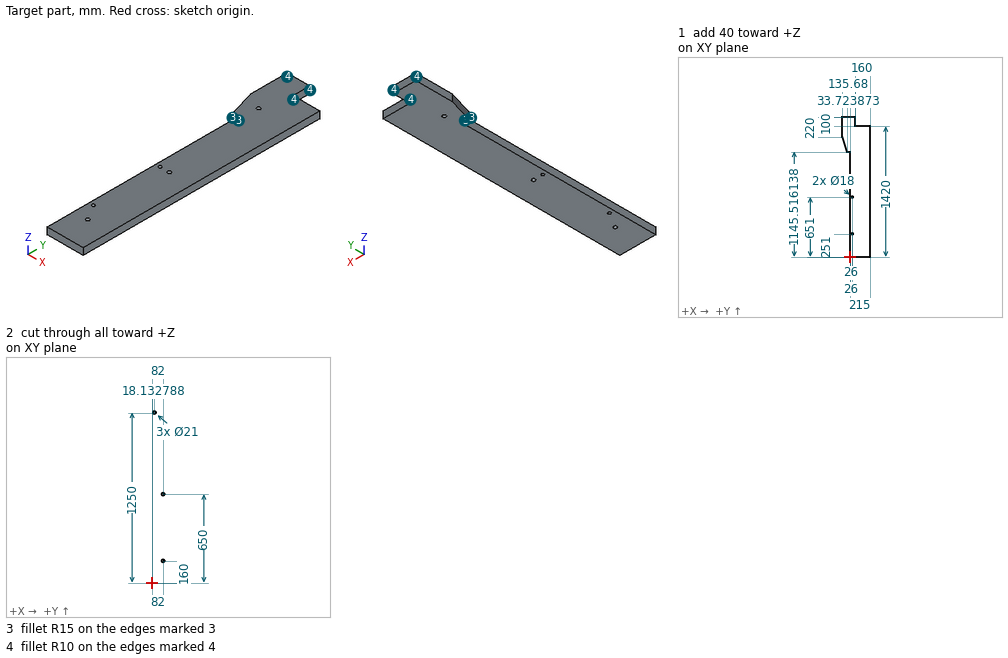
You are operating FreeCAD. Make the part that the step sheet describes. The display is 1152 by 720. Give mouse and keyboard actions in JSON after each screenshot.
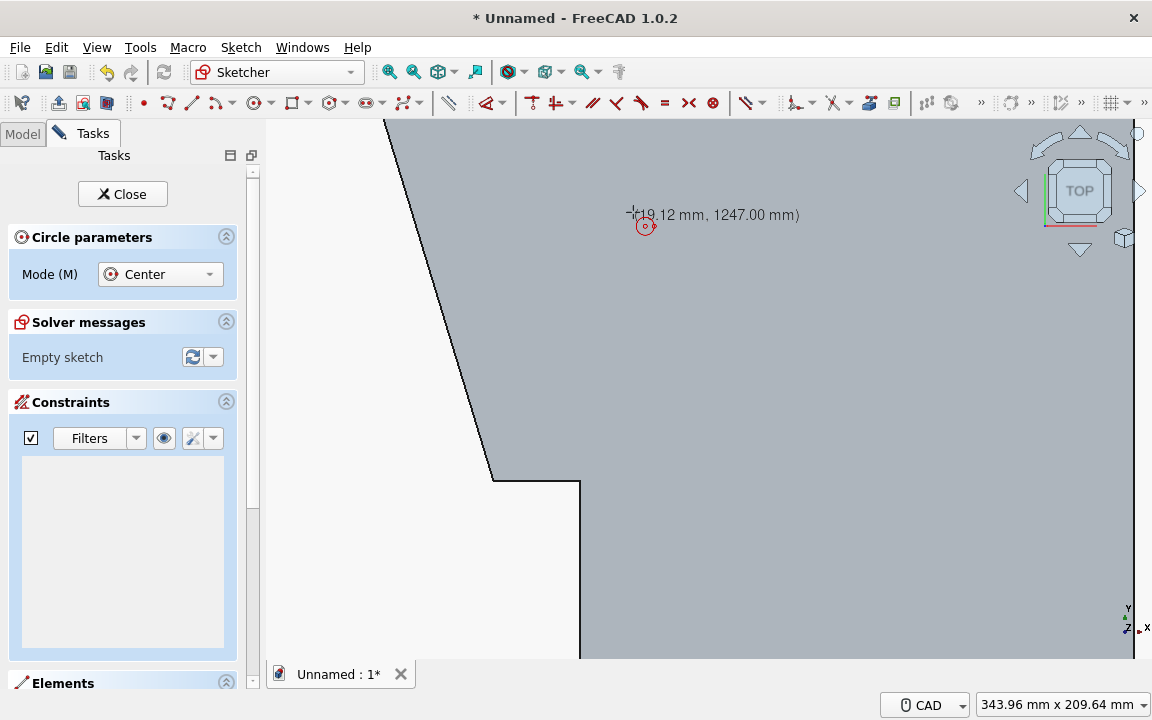
{"action": "scroll", "coordinate": [633, 212], "scroll_direction": "down", "scroll_amount": 11}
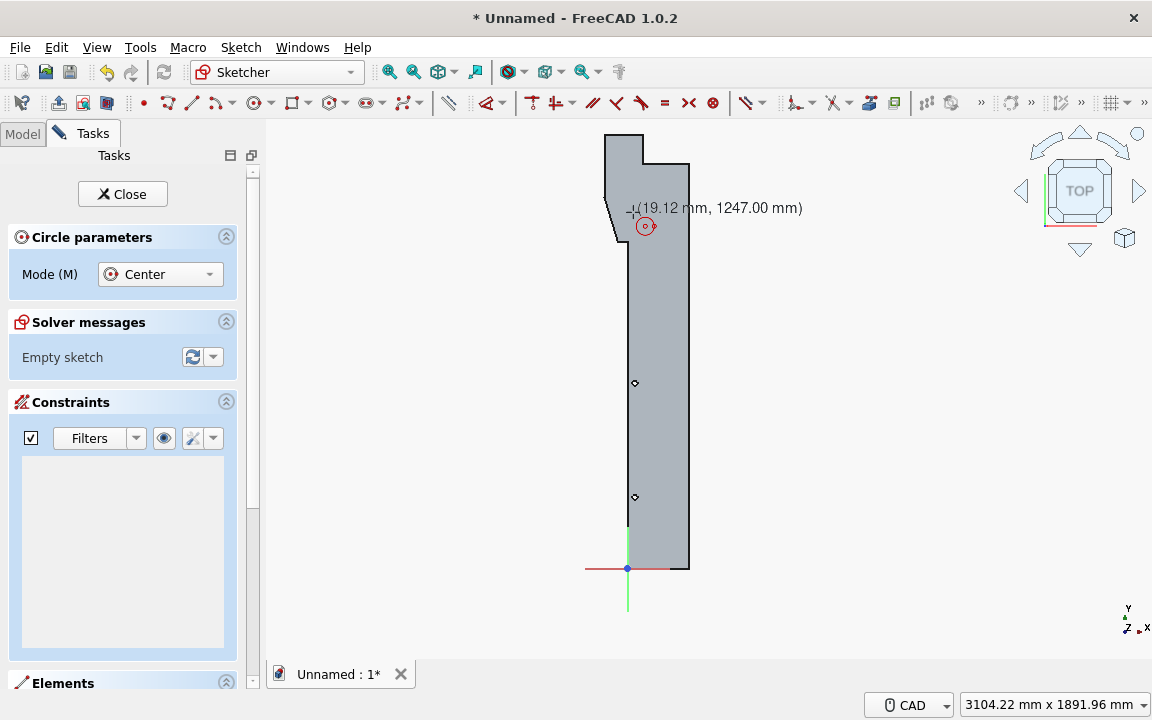
{"action": "scroll", "coordinate": [633, 212], "scroll_direction": "up", "scroll_amount": 6}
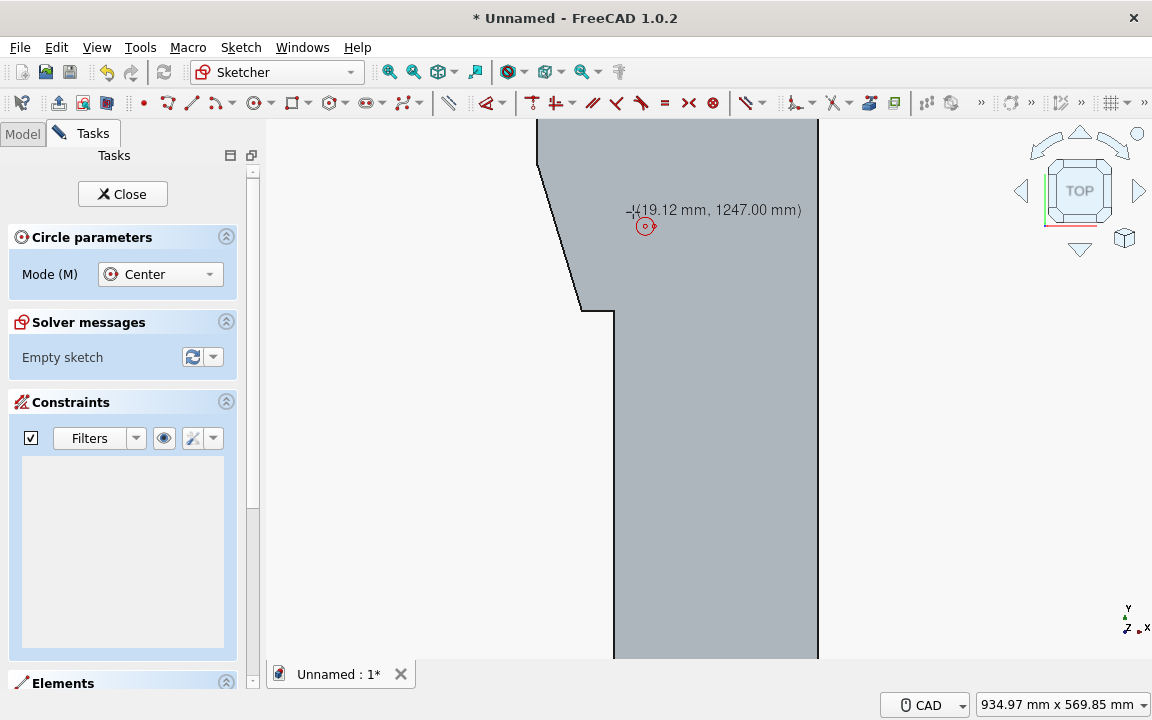
{"action": "left_click", "coordinate": [631, 212]}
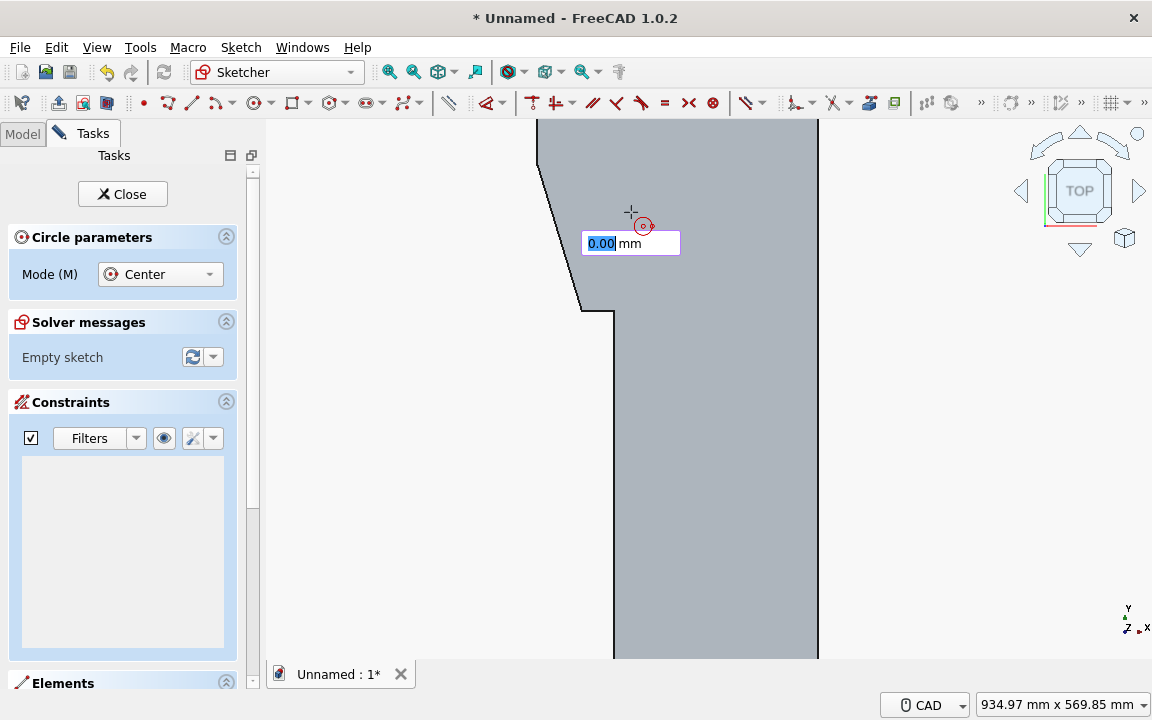
{"action": "scroll", "coordinate": [638, 205], "scroll_direction": "up", "scroll_amount": 3}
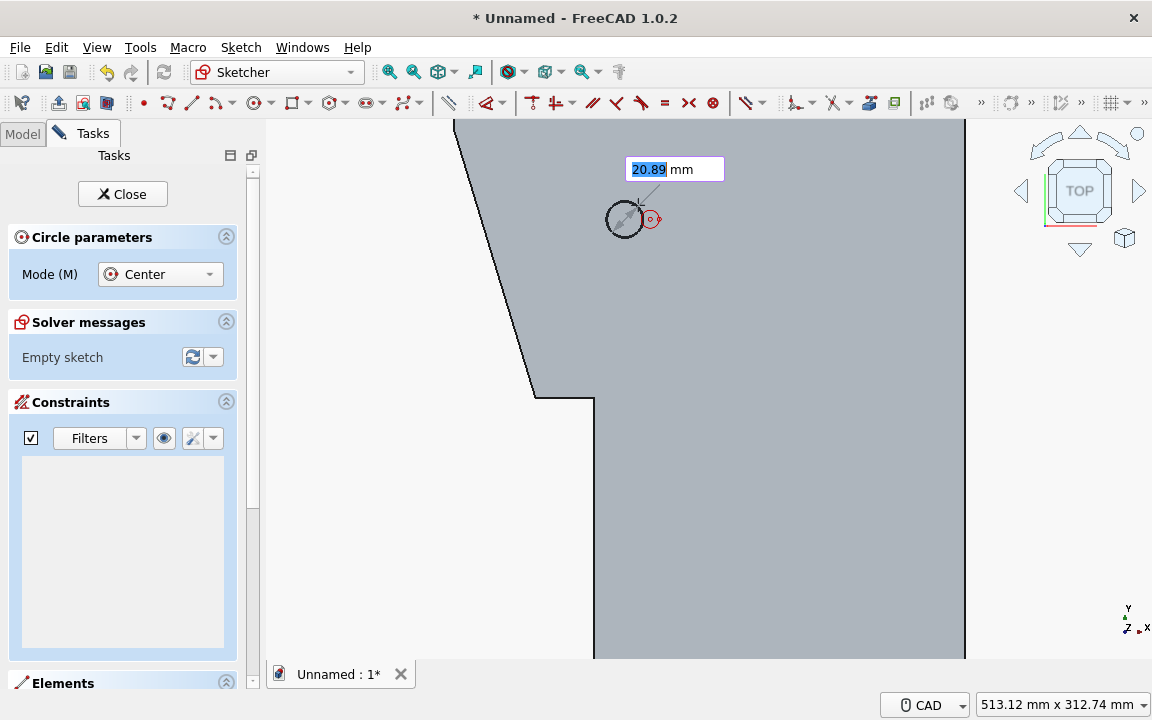
{"action": "left_click", "coordinate": [638, 205]}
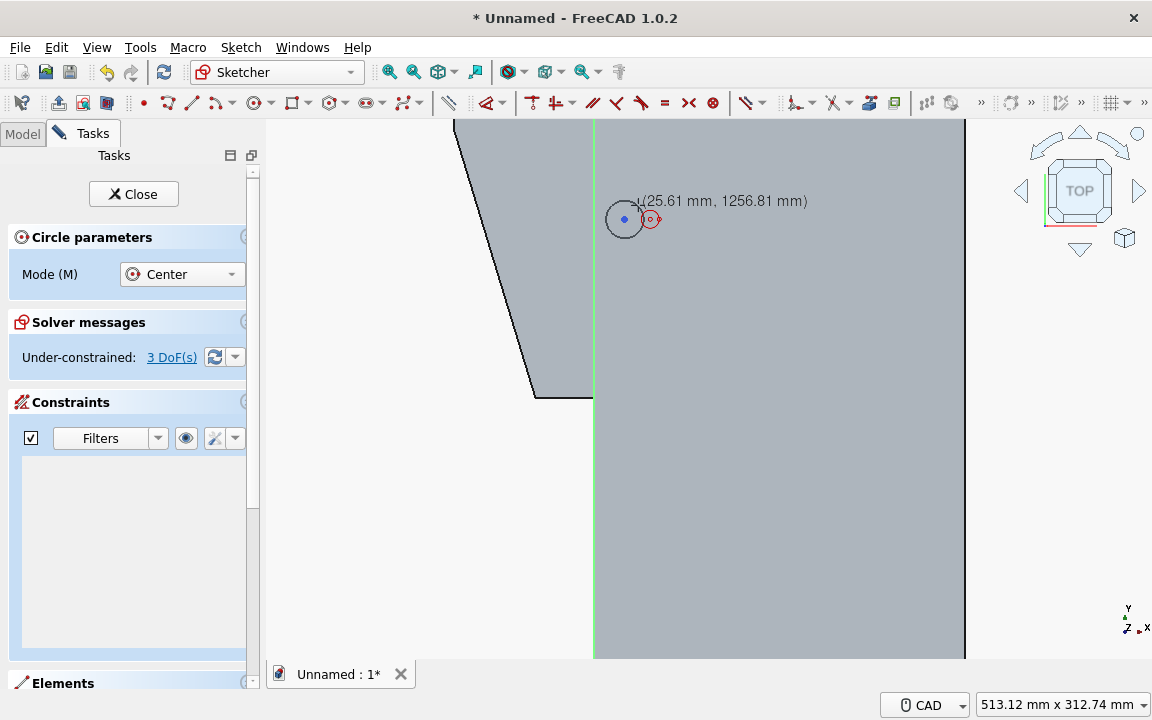
{"action": "scroll", "coordinate": [634, 211], "scroll_direction": "down", "scroll_amount": 9}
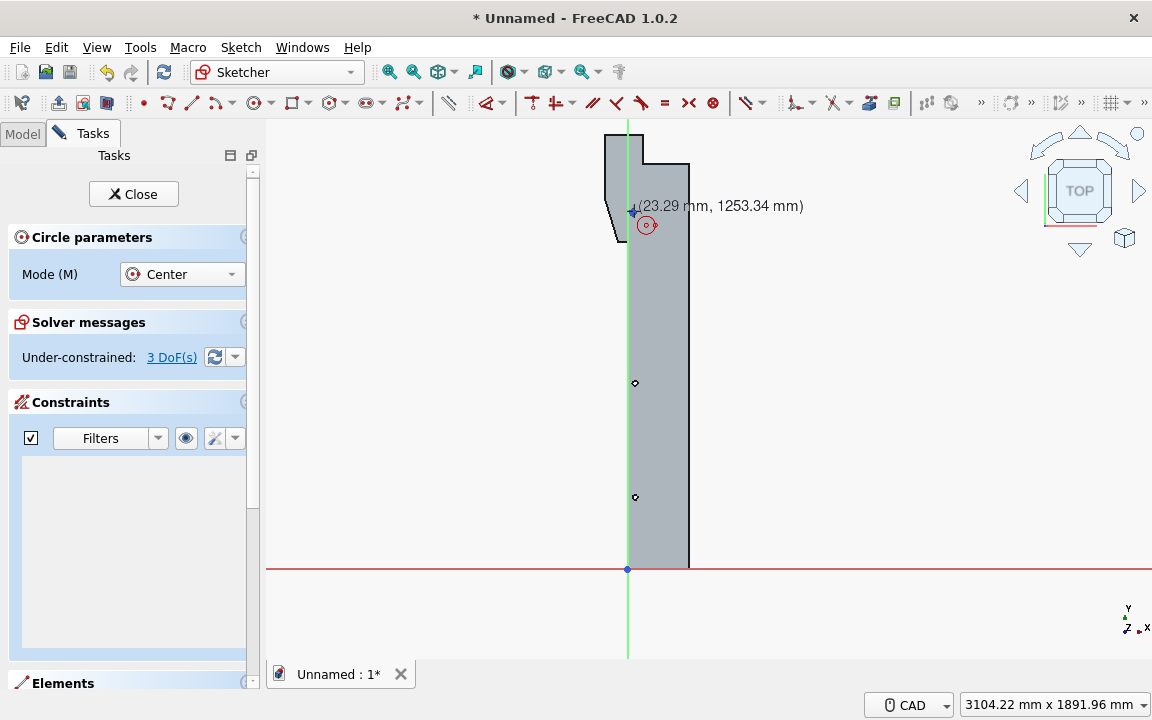
{"action": "scroll", "coordinate": [651, 384], "scroll_direction": "up", "scroll_amount": 11}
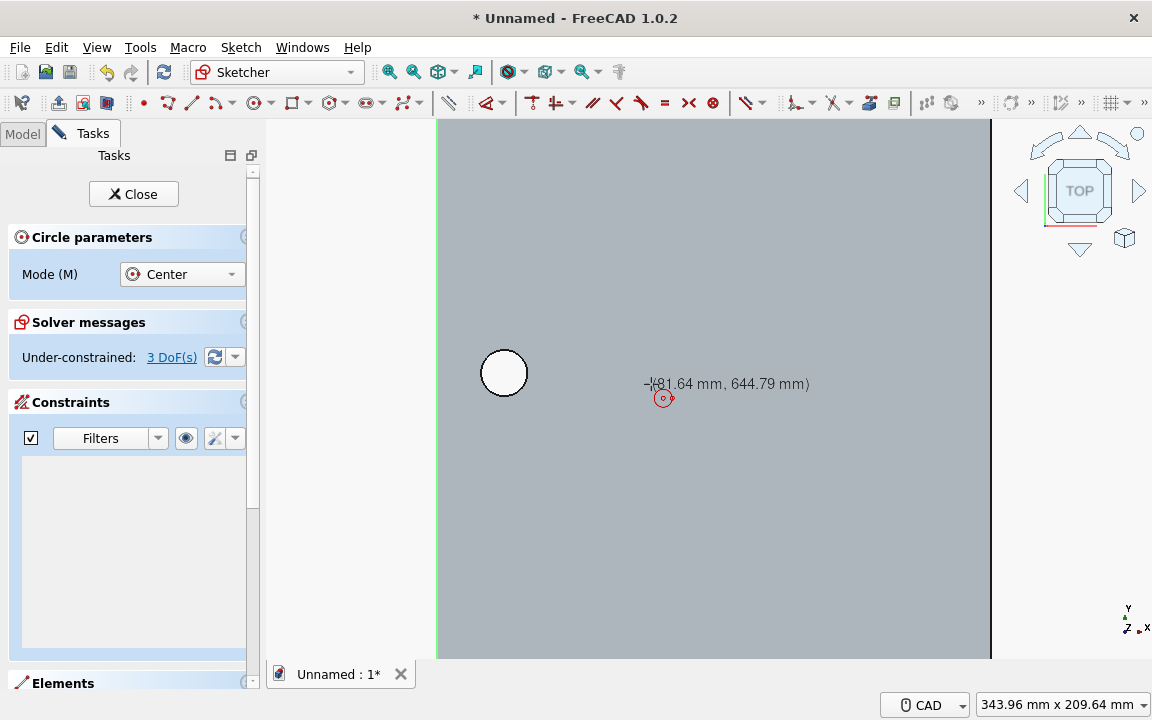
{"action": "scroll", "coordinate": [651, 384], "scroll_direction": "down", "scroll_amount": 11}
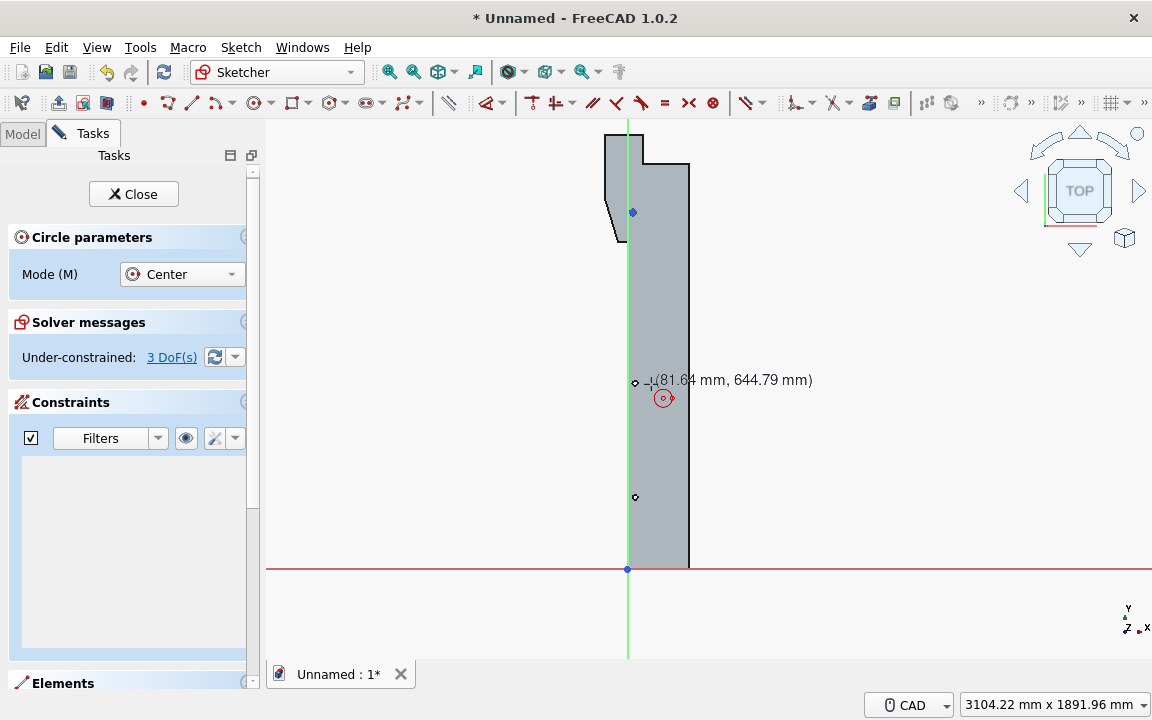
{"action": "left_click", "coordinate": [651, 384]}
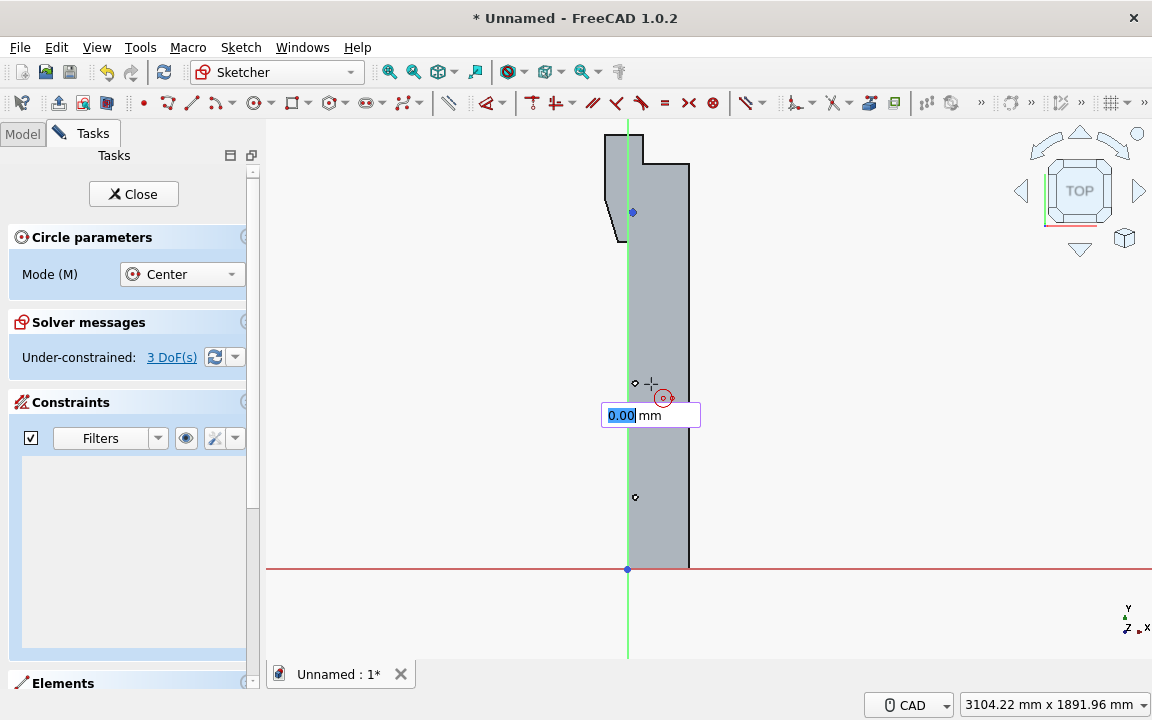
{"action": "scroll", "coordinate": [653, 381], "scroll_direction": "up", "scroll_amount": 9}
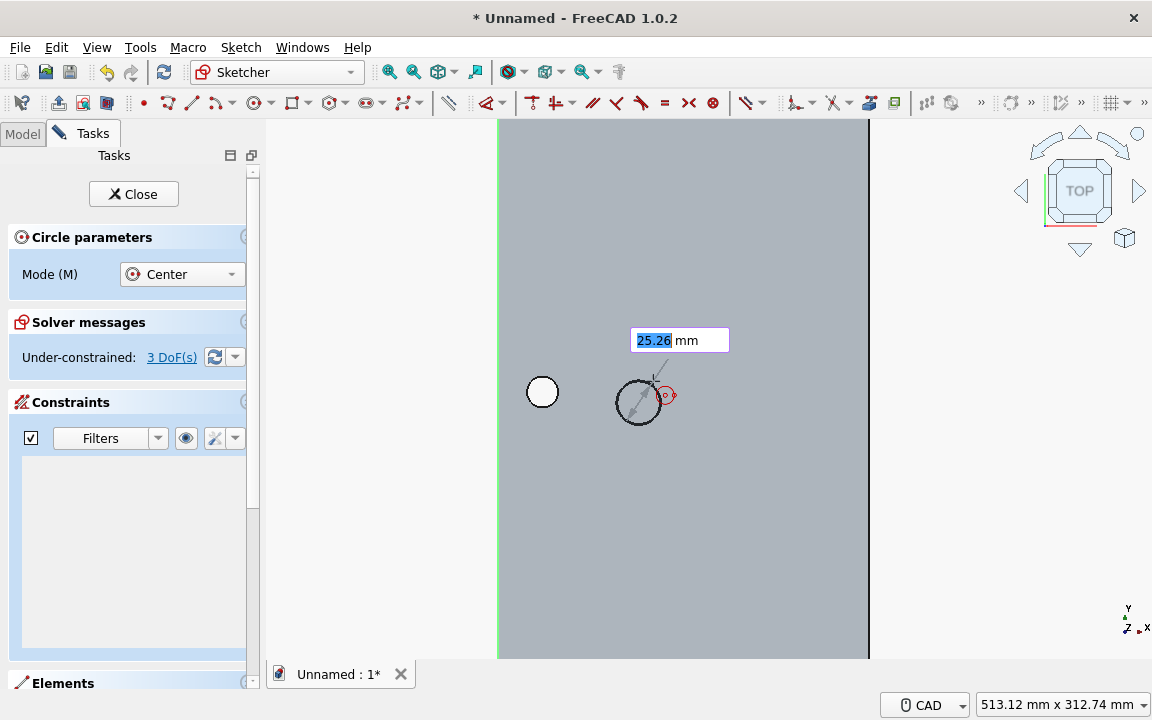
{"action": "left_click", "coordinate": [652, 381]}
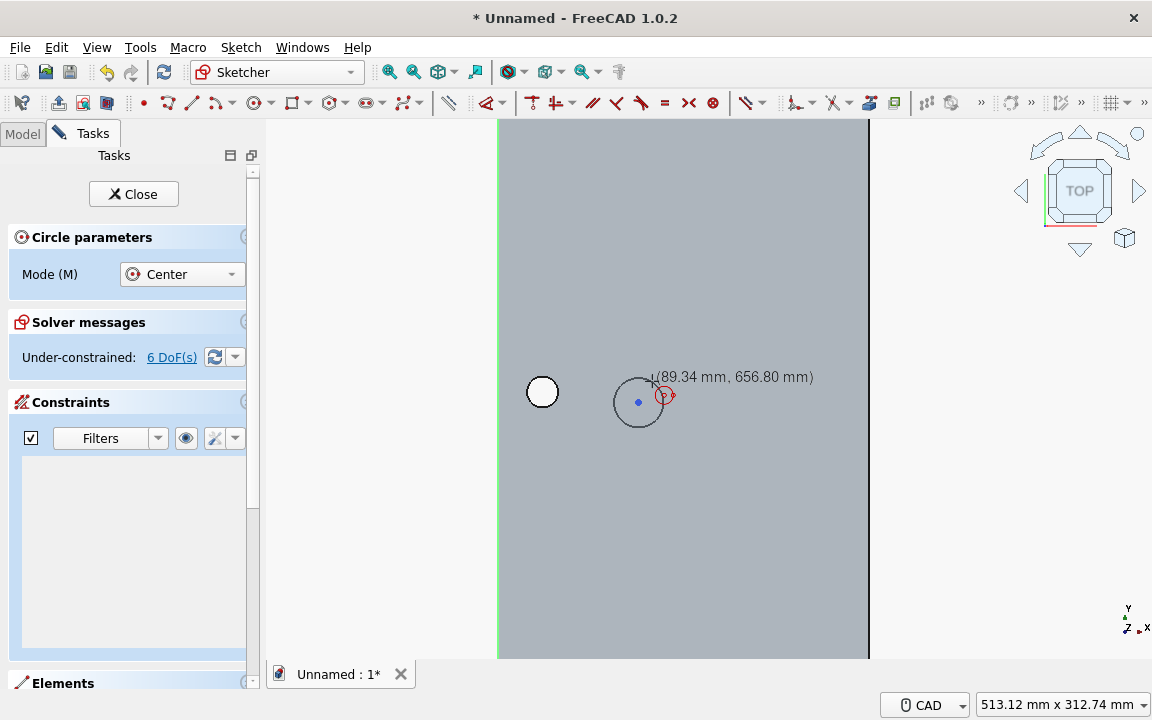
{"action": "scroll", "coordinate": [653, 381], "scroll_direction": "down", "scroll_amount": 9}